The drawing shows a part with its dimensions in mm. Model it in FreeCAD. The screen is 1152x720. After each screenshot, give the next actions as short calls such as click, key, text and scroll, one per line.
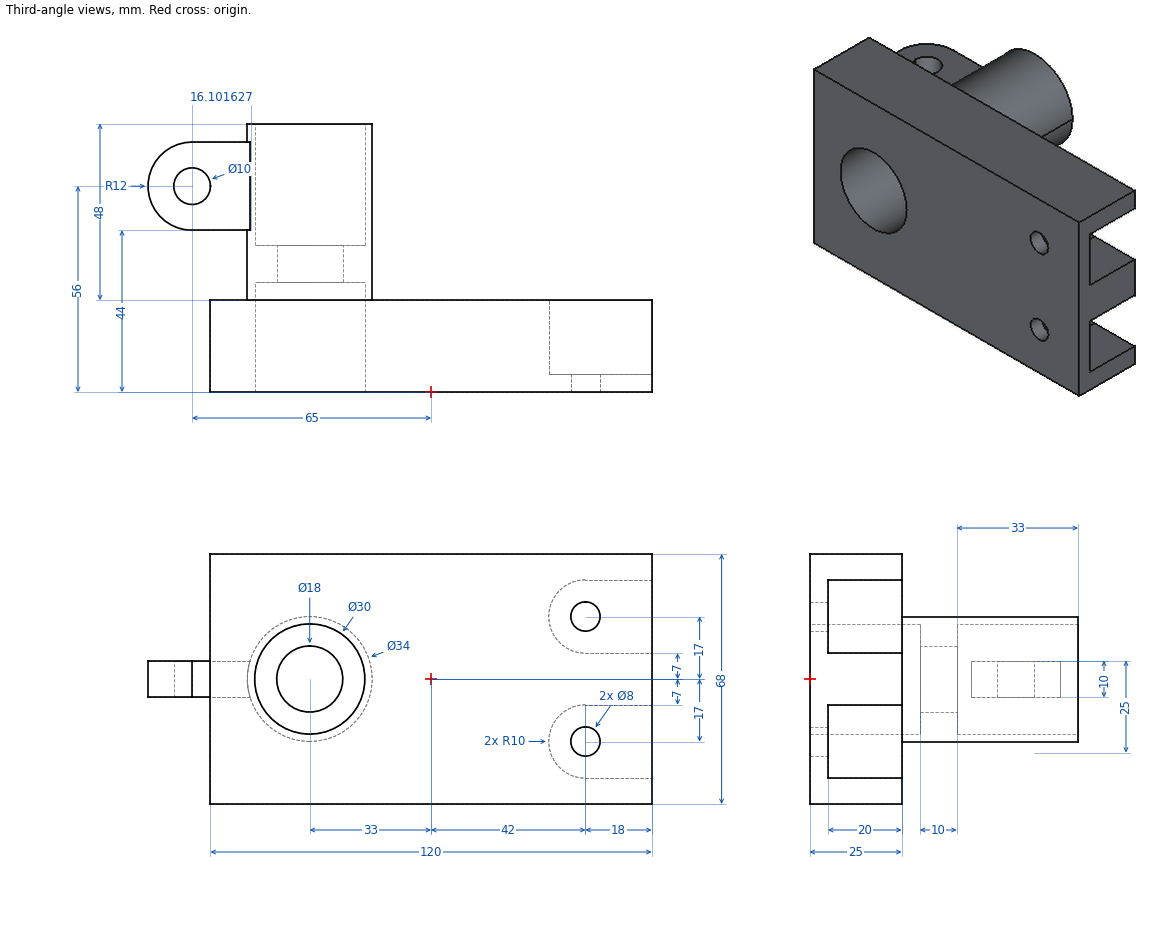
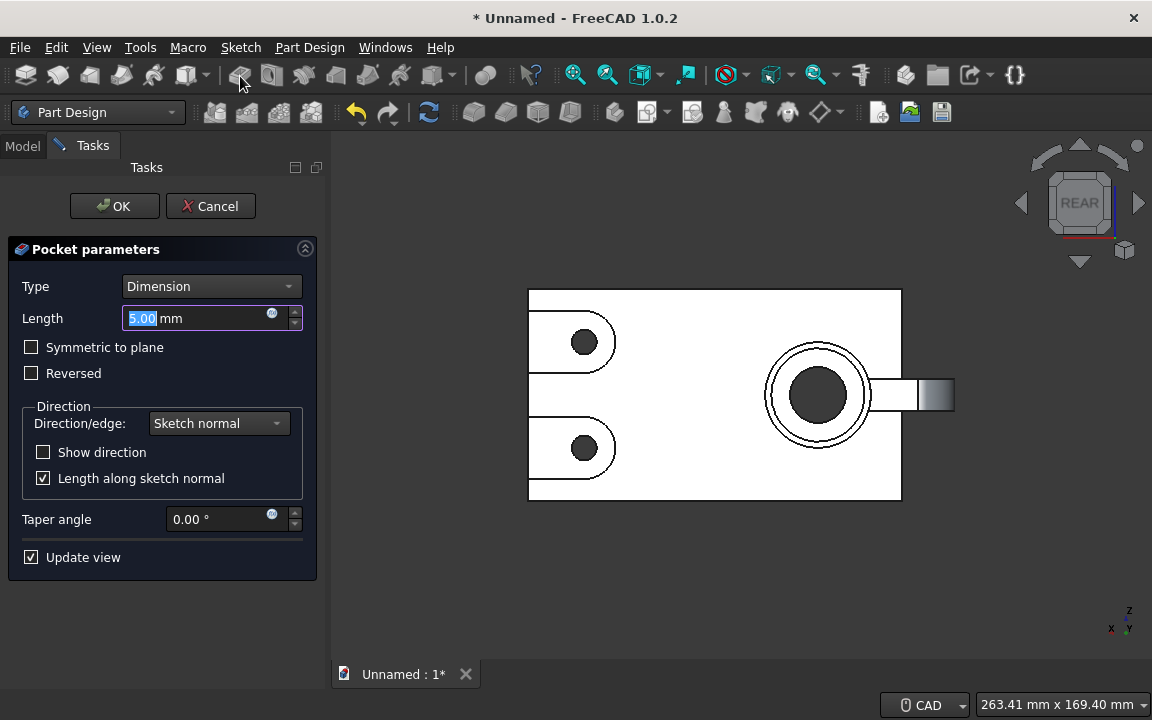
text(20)
key(Tab)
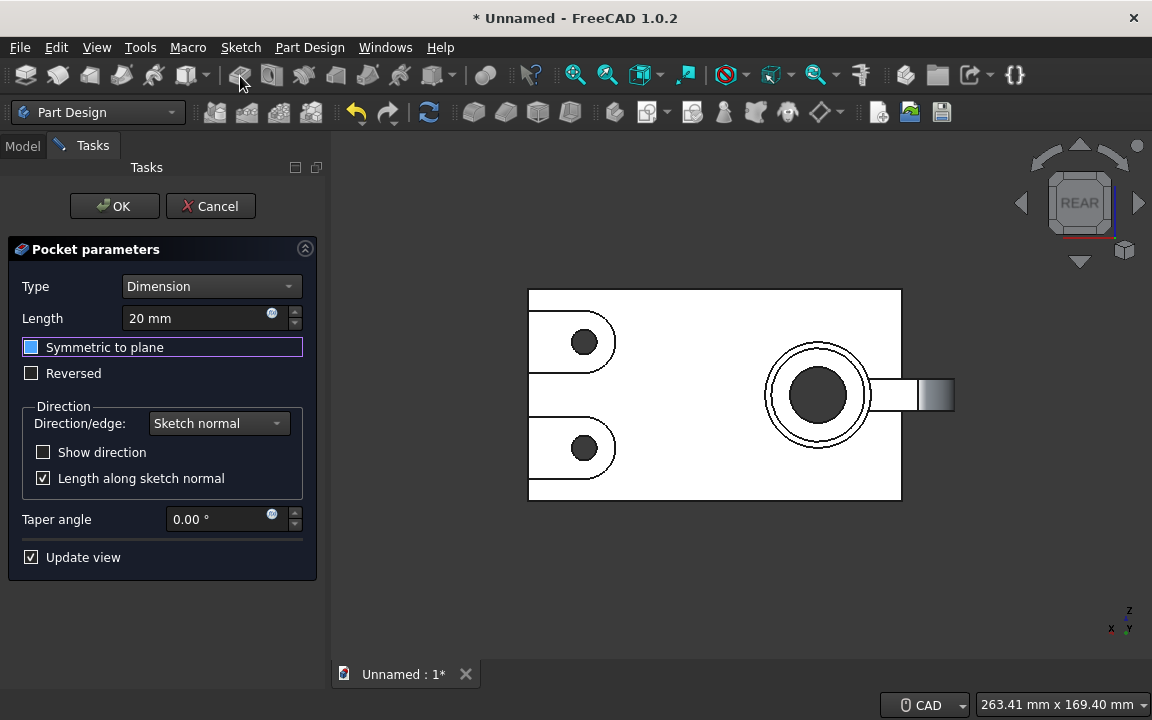
click(115, 206)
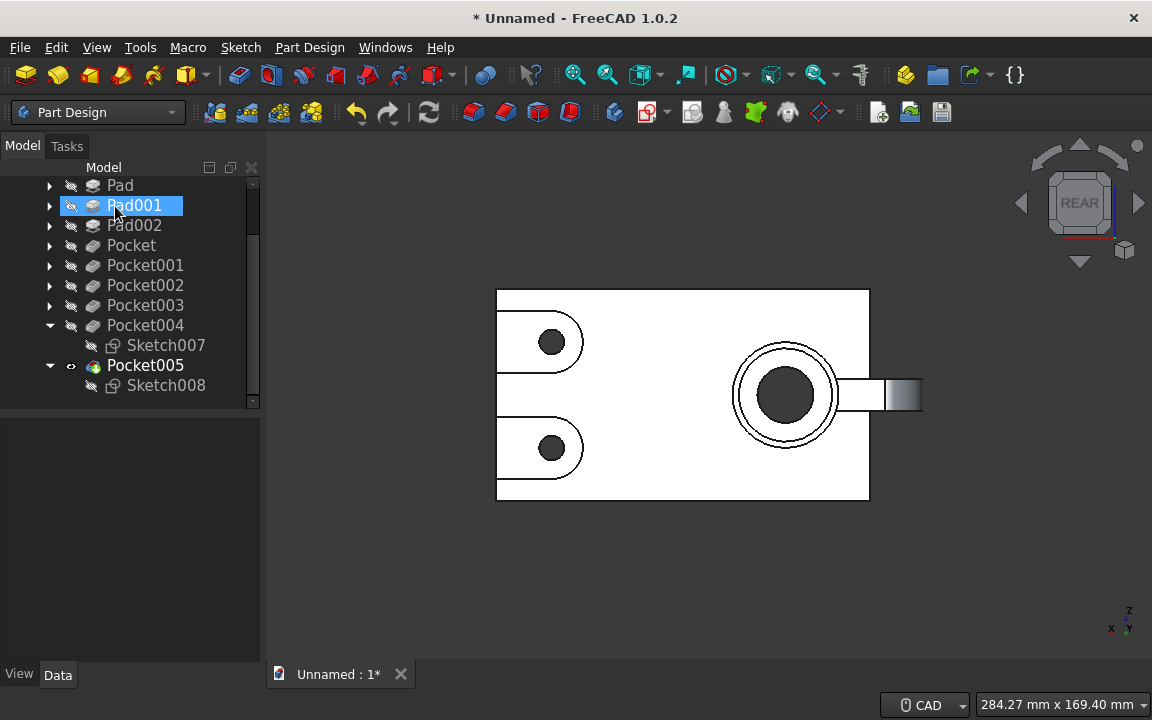
key(0)